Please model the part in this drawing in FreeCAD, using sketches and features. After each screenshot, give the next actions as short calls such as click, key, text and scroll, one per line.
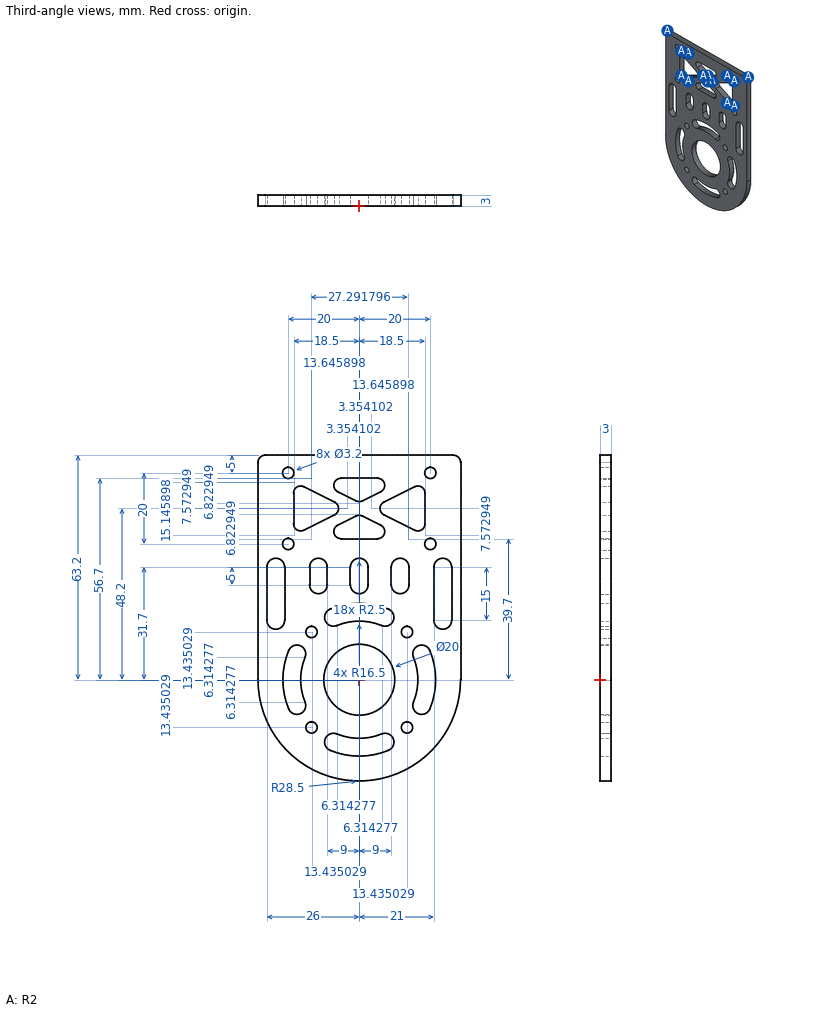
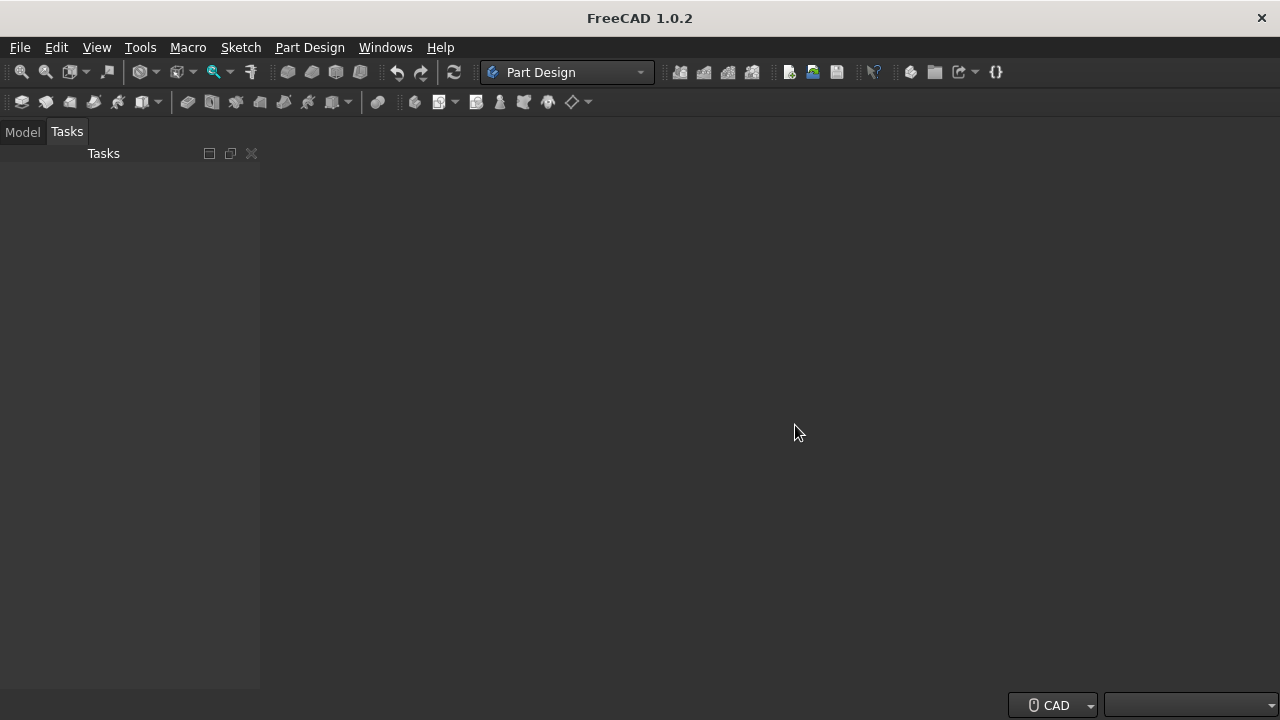
click(790, 72)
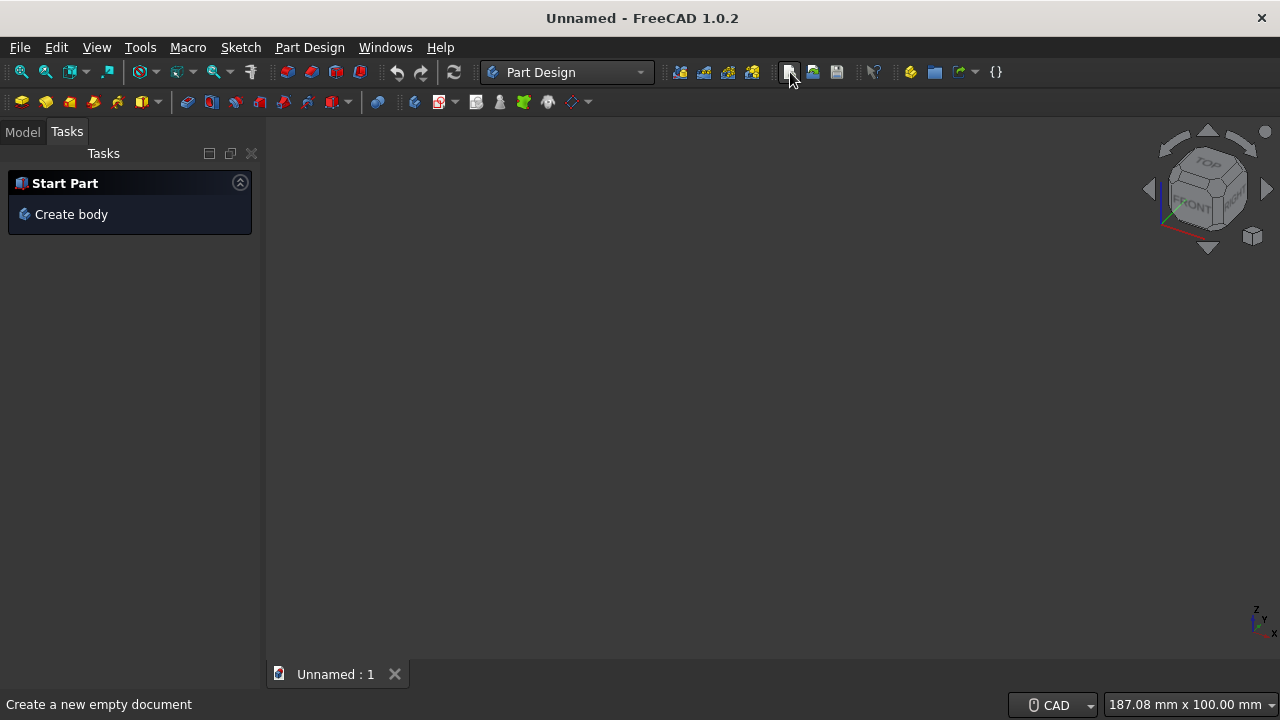
click(440, 102)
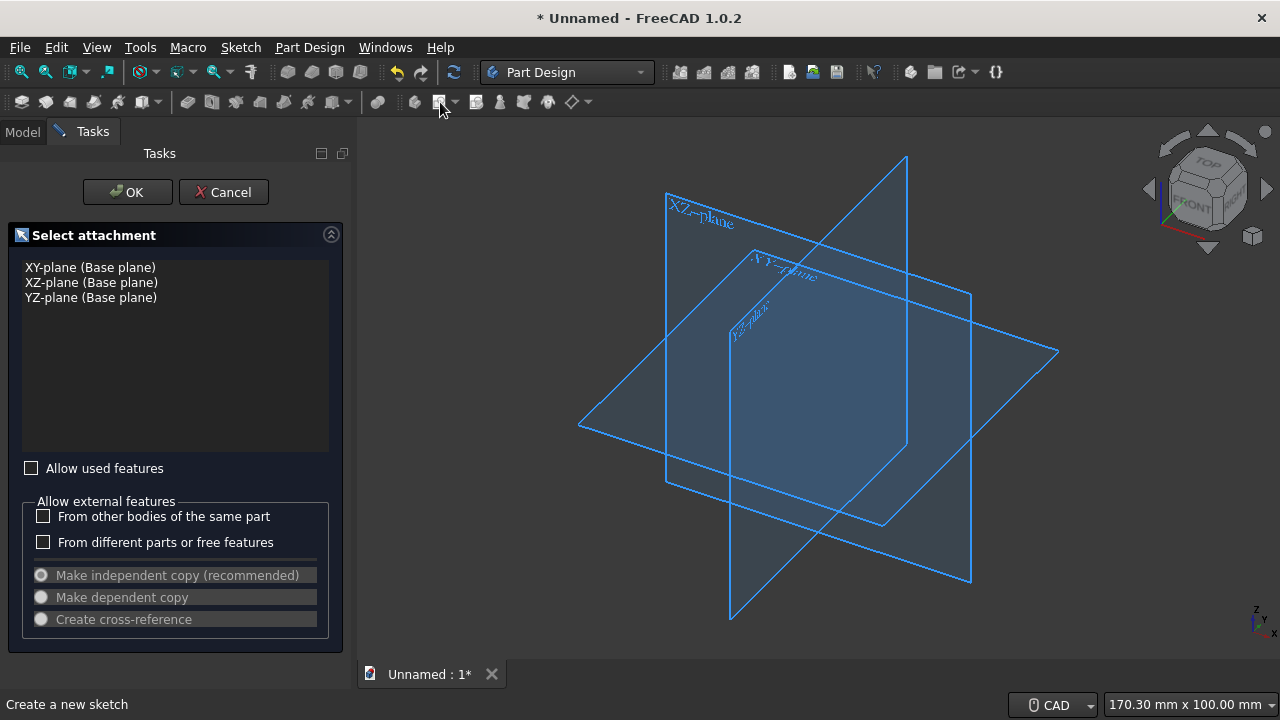
click(82, 282)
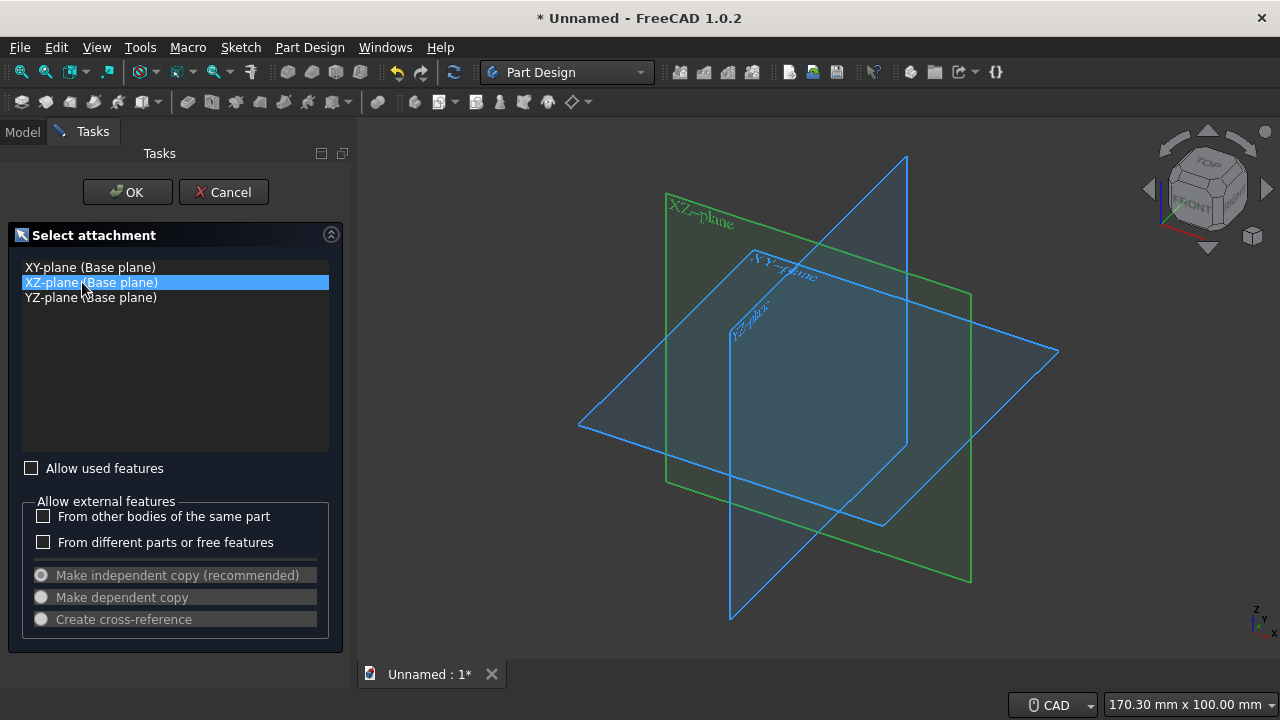
click(128, 192)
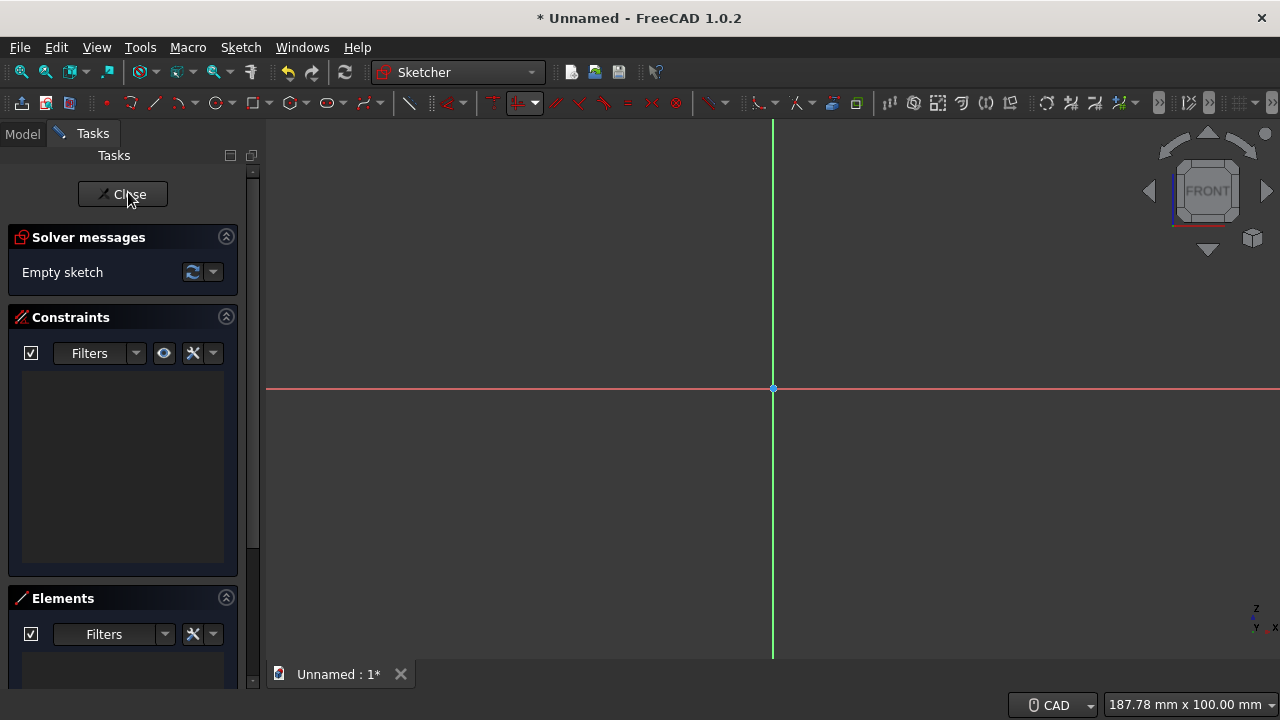
scroll(565, 579, down, 2)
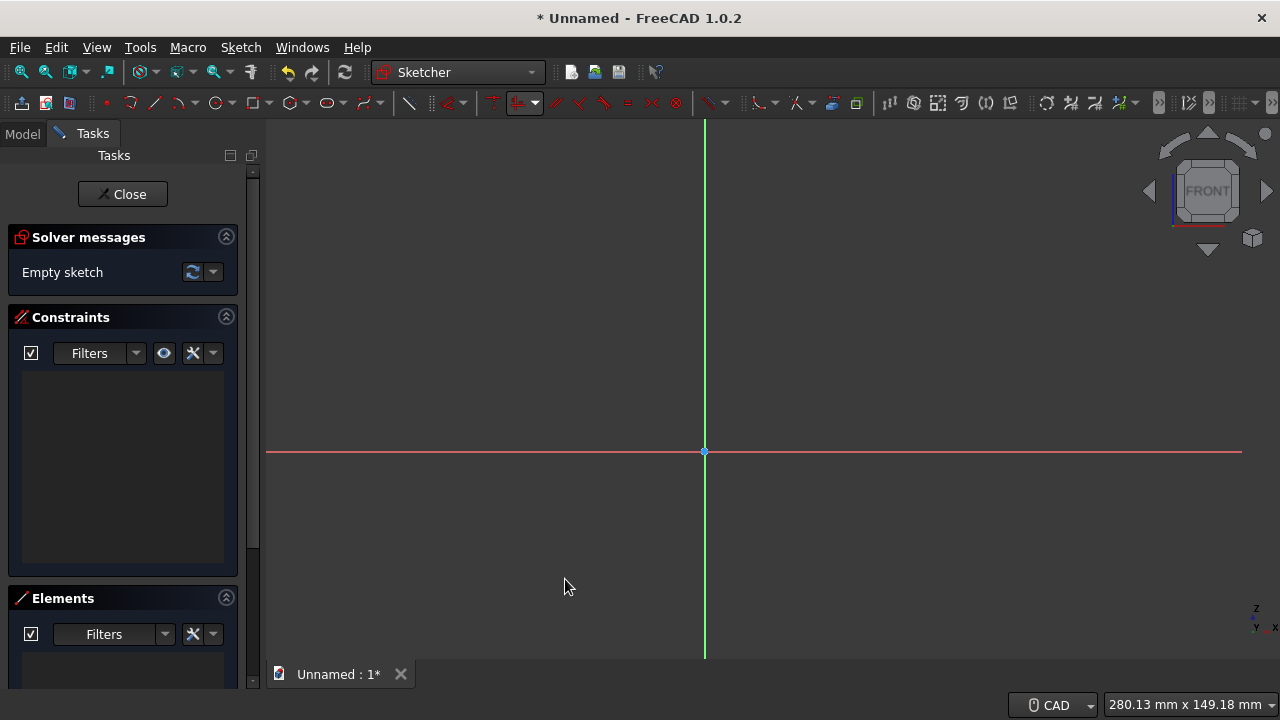
click(132, 104)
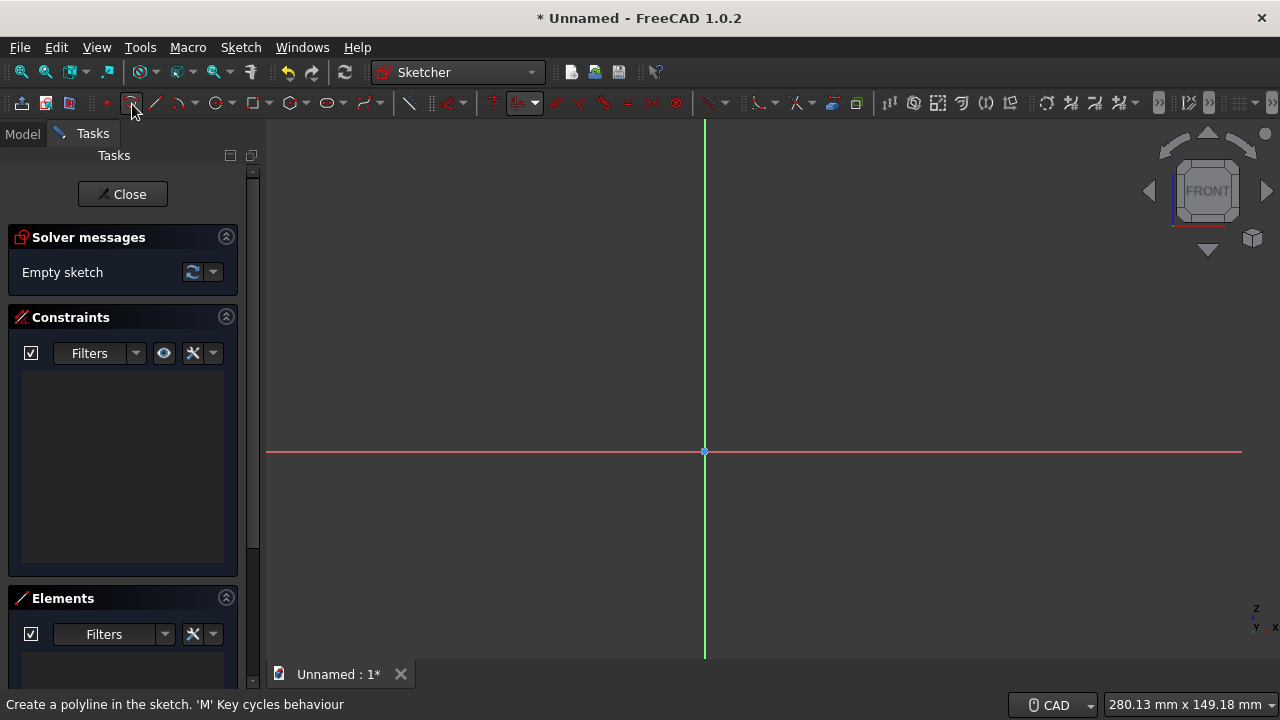
click(601, 452)
click(601, 223)
click(808, 223)
click(808, 452)
right_click(808, 452)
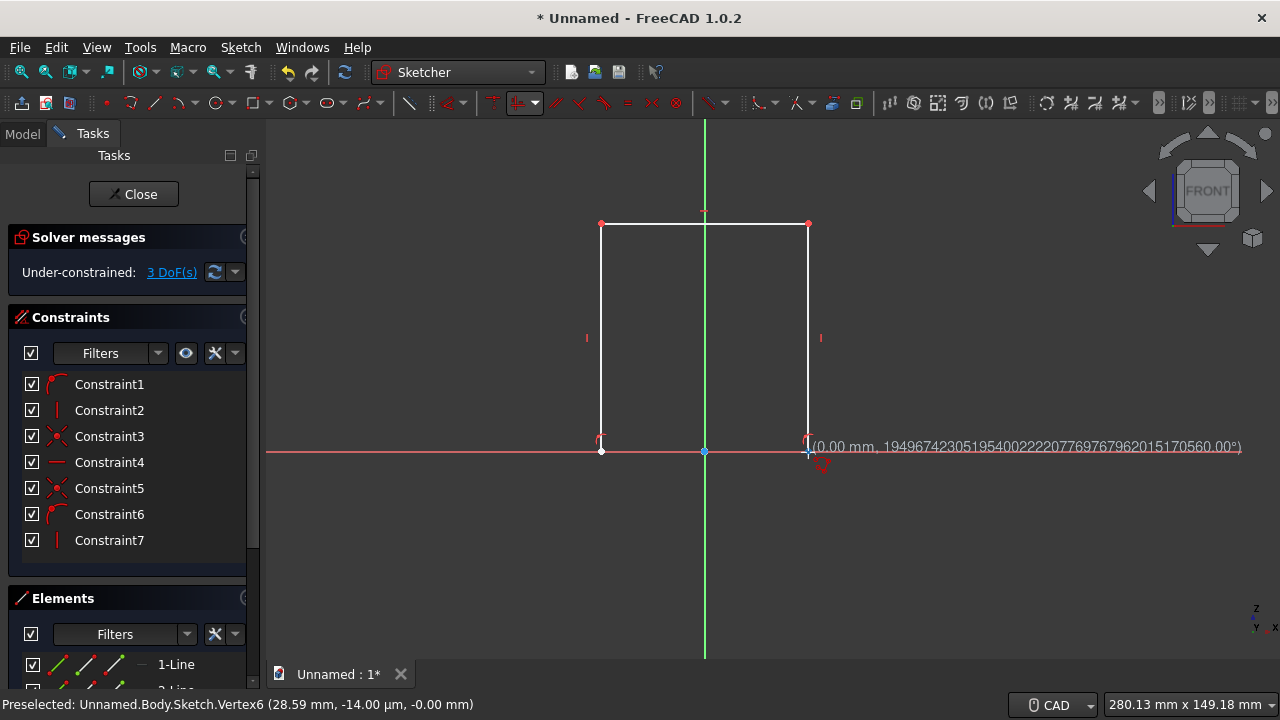
key(g)
key(3)
key(a)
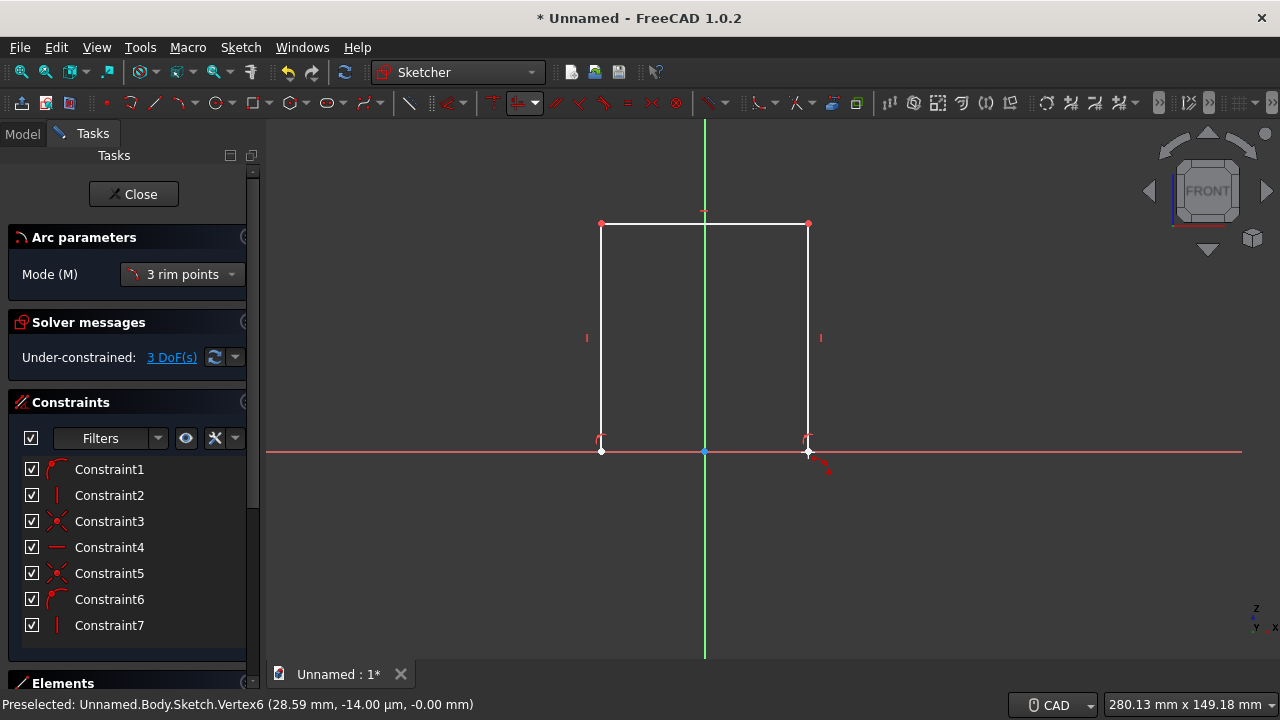
click(808, 452)
click(601, 452)
click(673, 550)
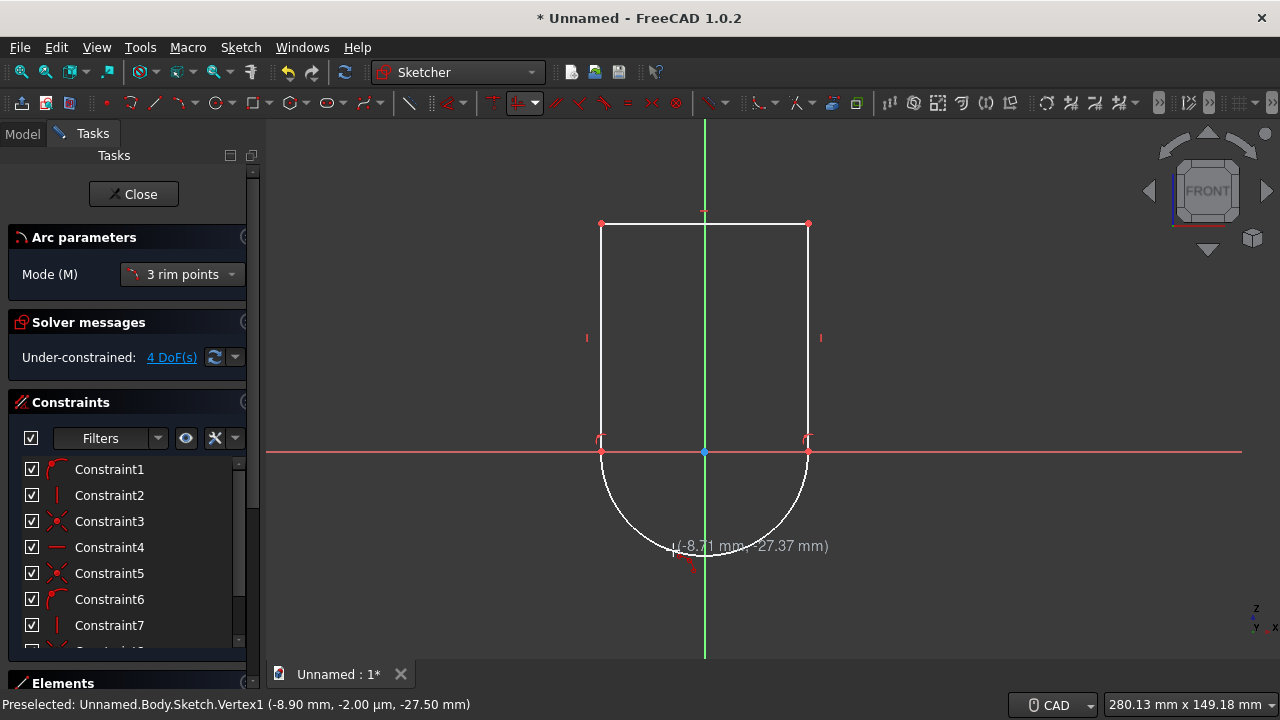
key(g)
key(c)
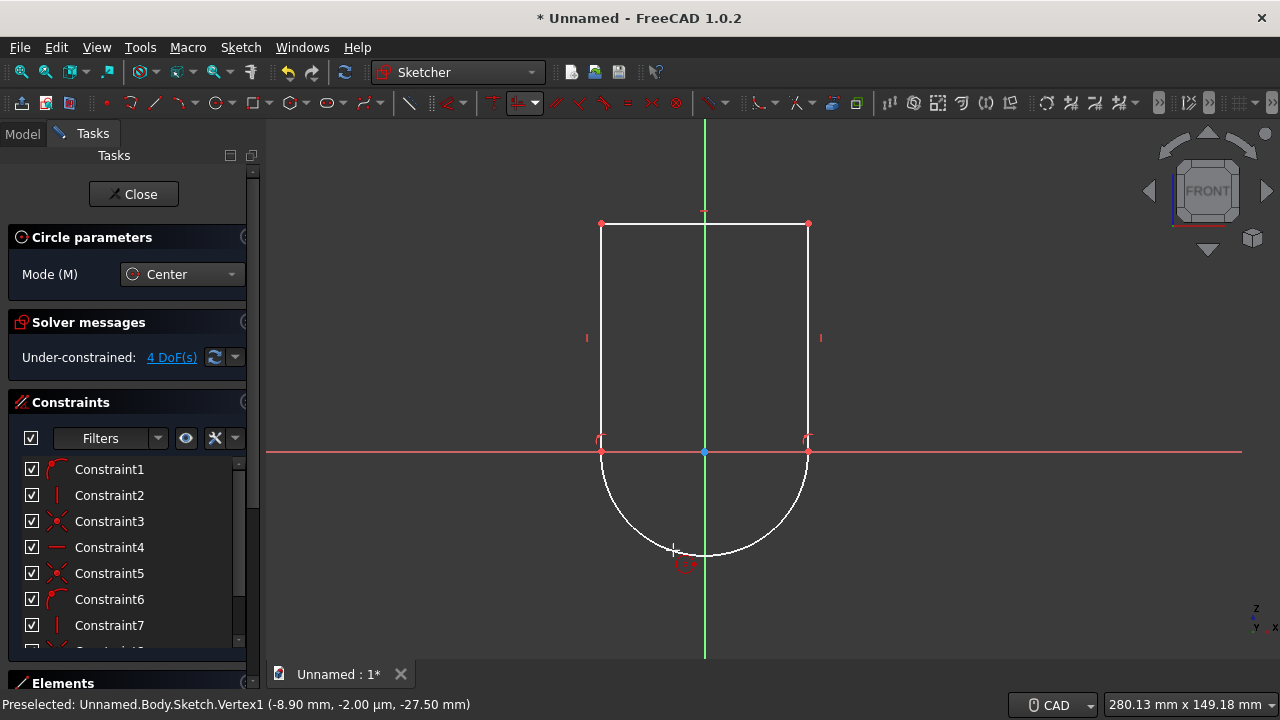
scroll(632, 241, up, 7)